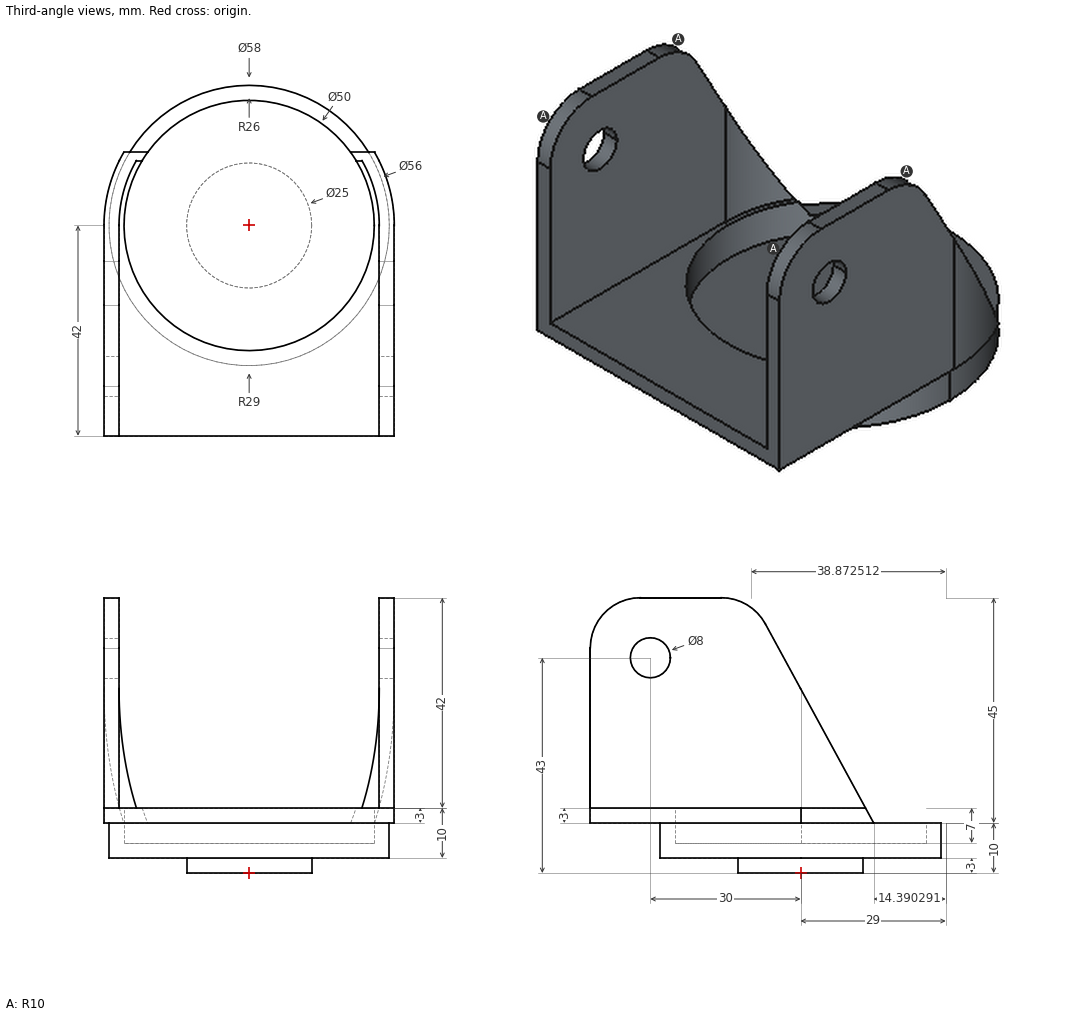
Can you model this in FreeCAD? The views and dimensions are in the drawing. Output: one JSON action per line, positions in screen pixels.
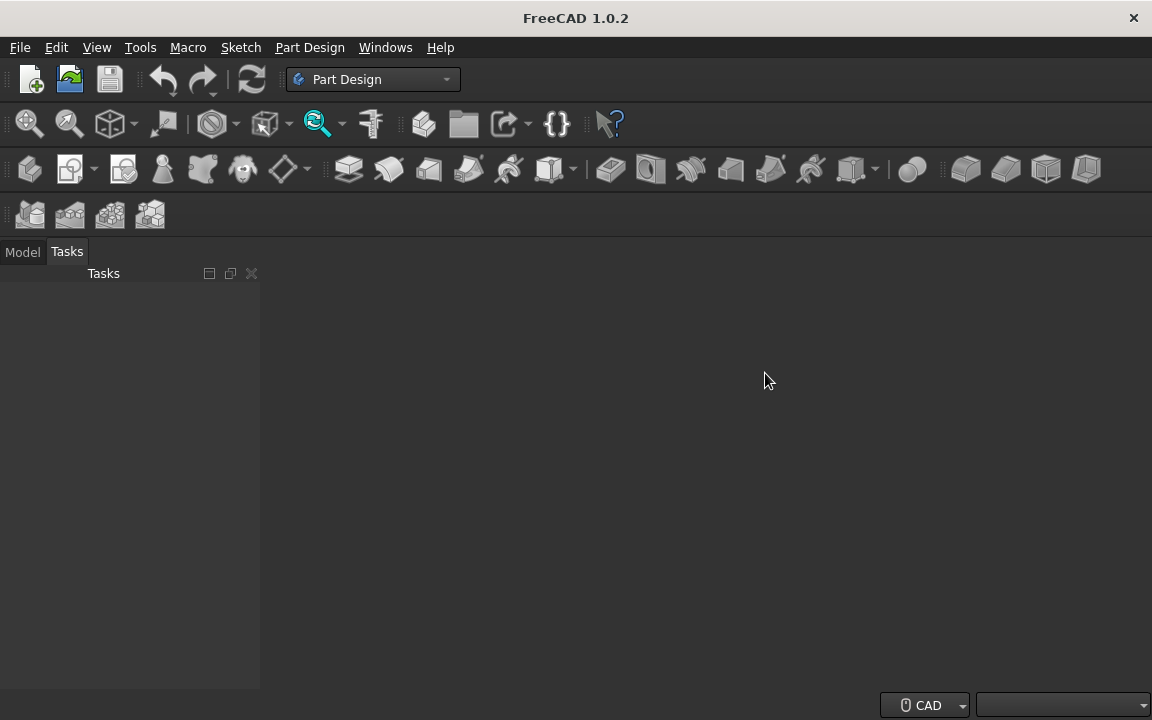
{"action": "left_click", "coordinate": [30, 80]}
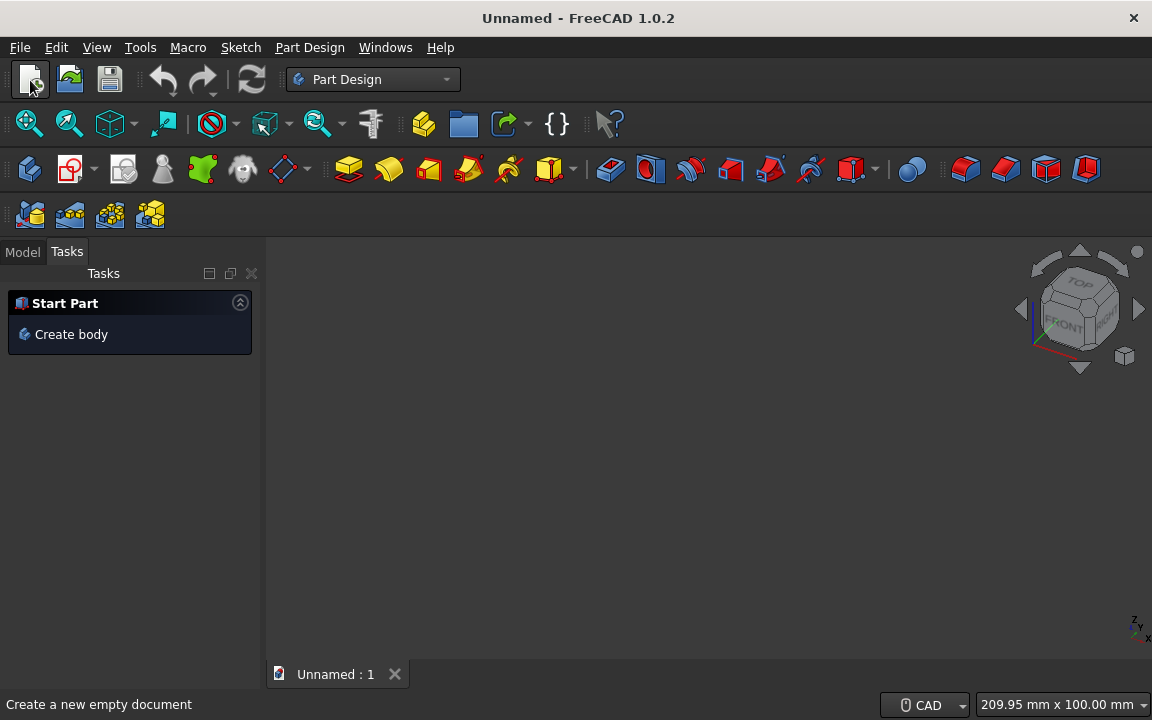
{"action": "left_click", "coordinate": [70, 170]}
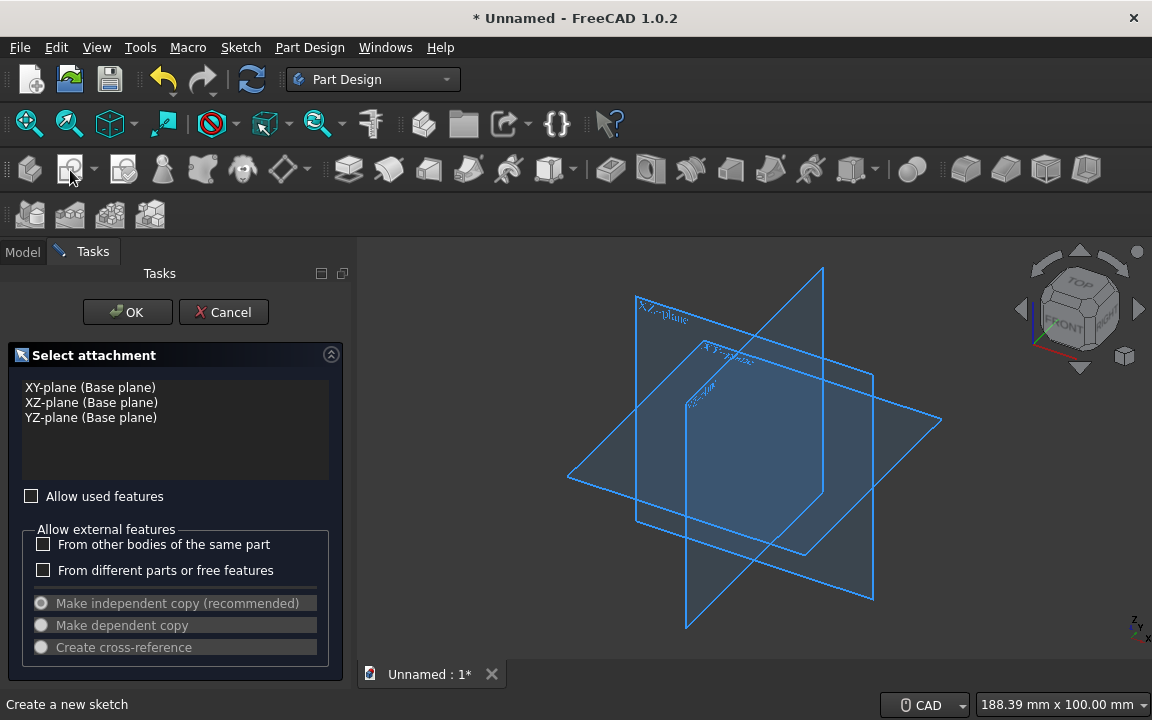
{"action": "left_click", "coordinate": [82, 388]}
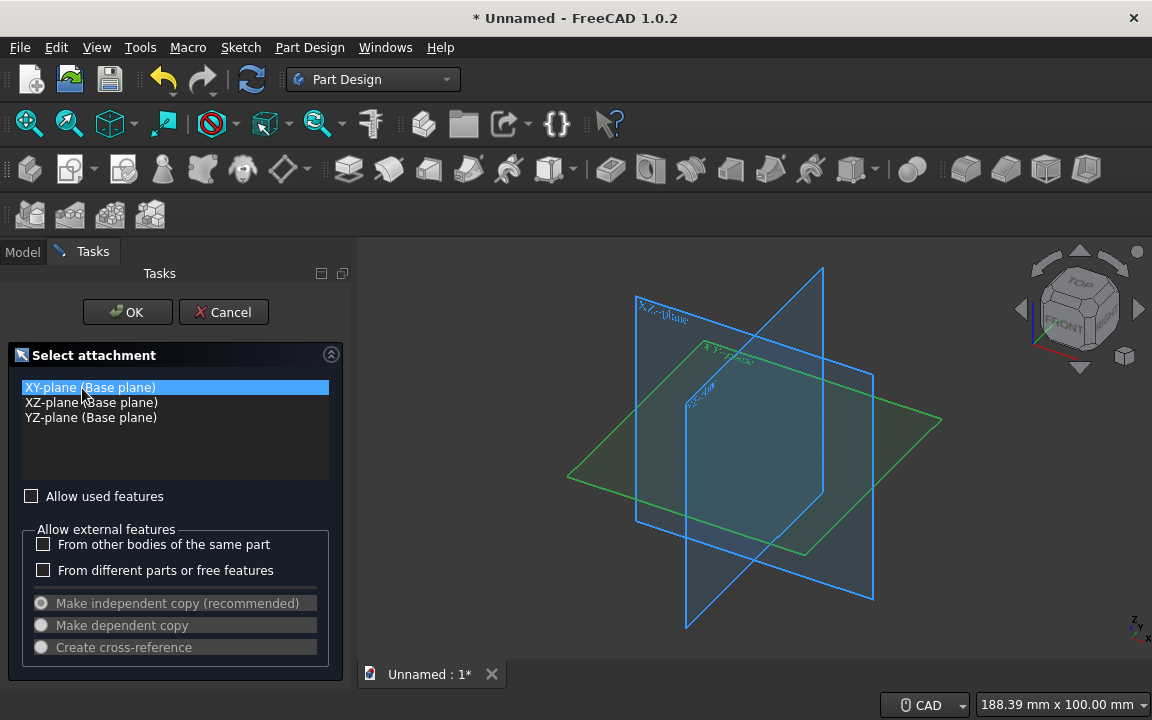
{"action": "left_click", "coordinate": [128, 312]}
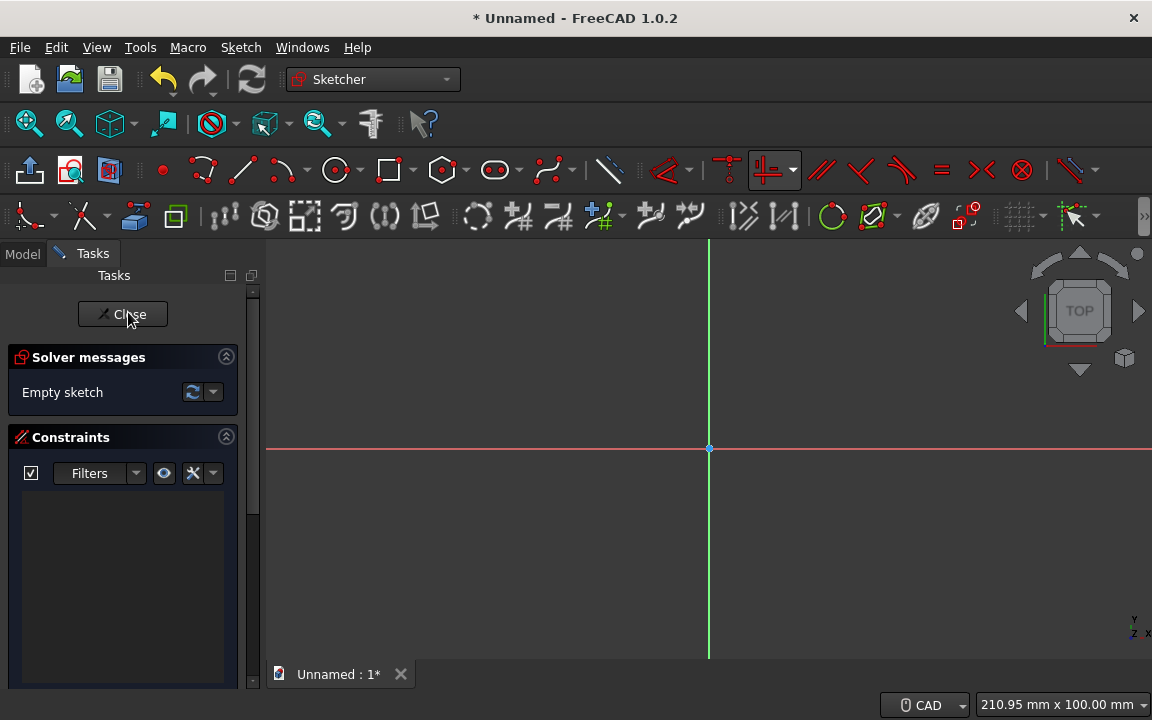
{"action": "scroll", "coordinate": [765, 449], "scroll_direction": "up", "scroll_amount": 4}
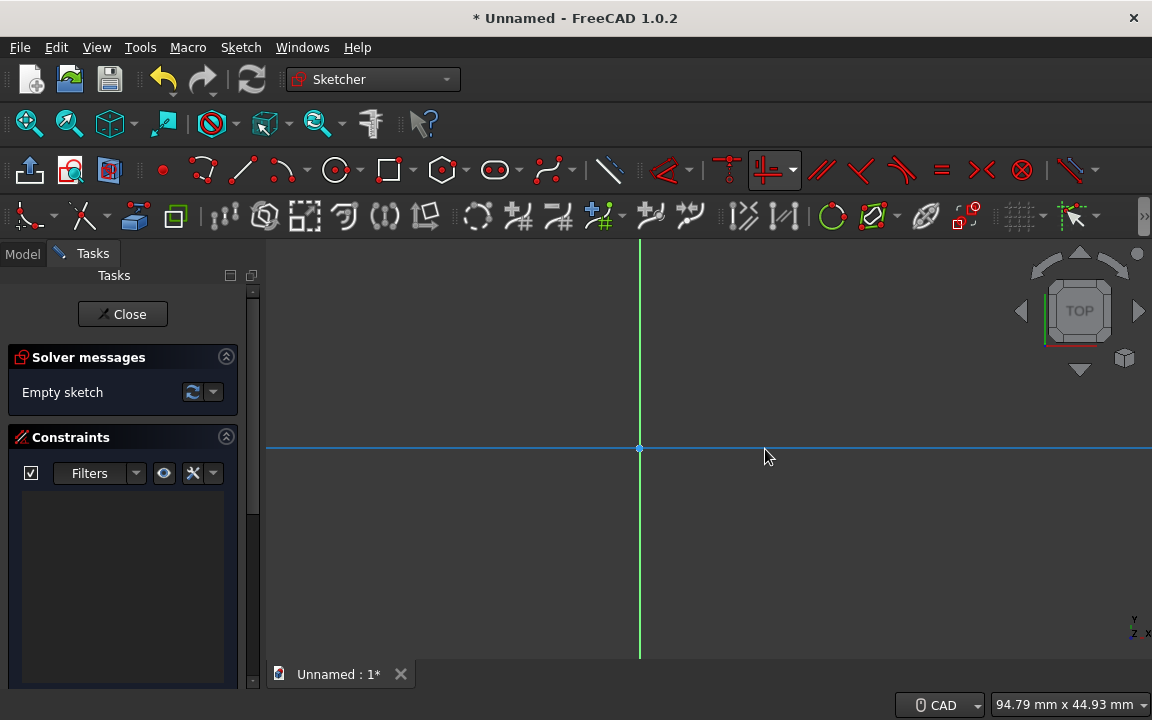
{"action": "left_click", "coordinate": [336, 170]}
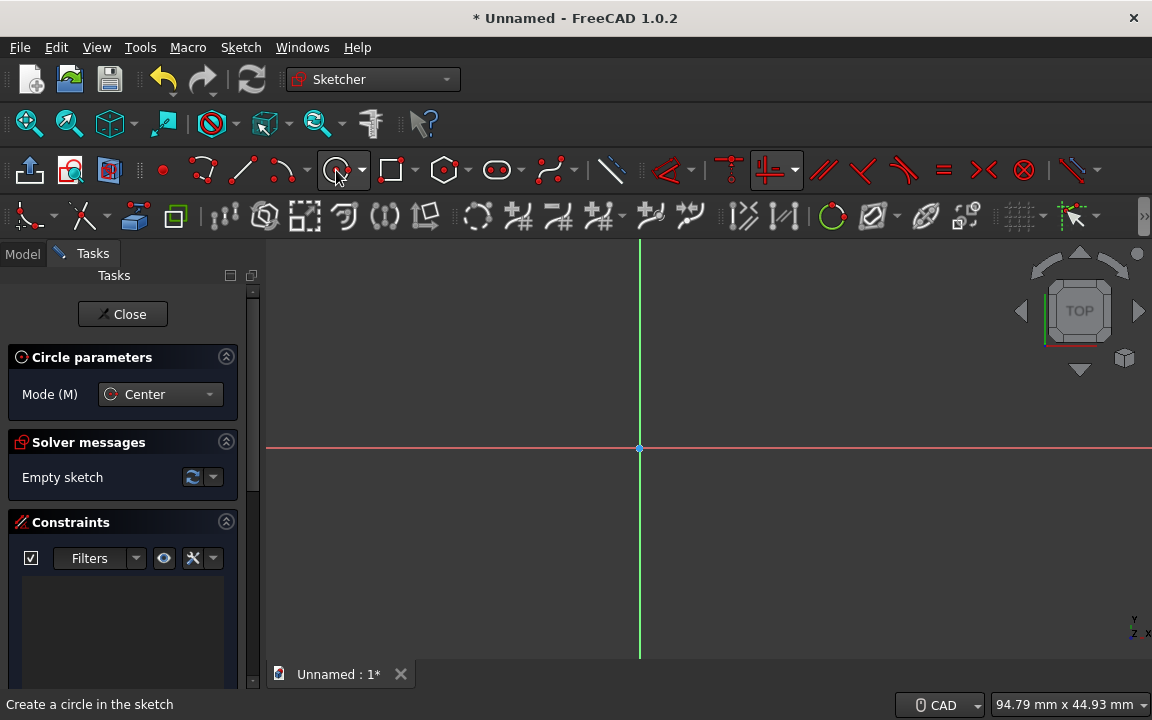
{"action": "left_click", "coordinate": [640, 448]}
{"action": "left_click", "coordinate": [722, 366]}
{"action": "key", "text": "Escape"}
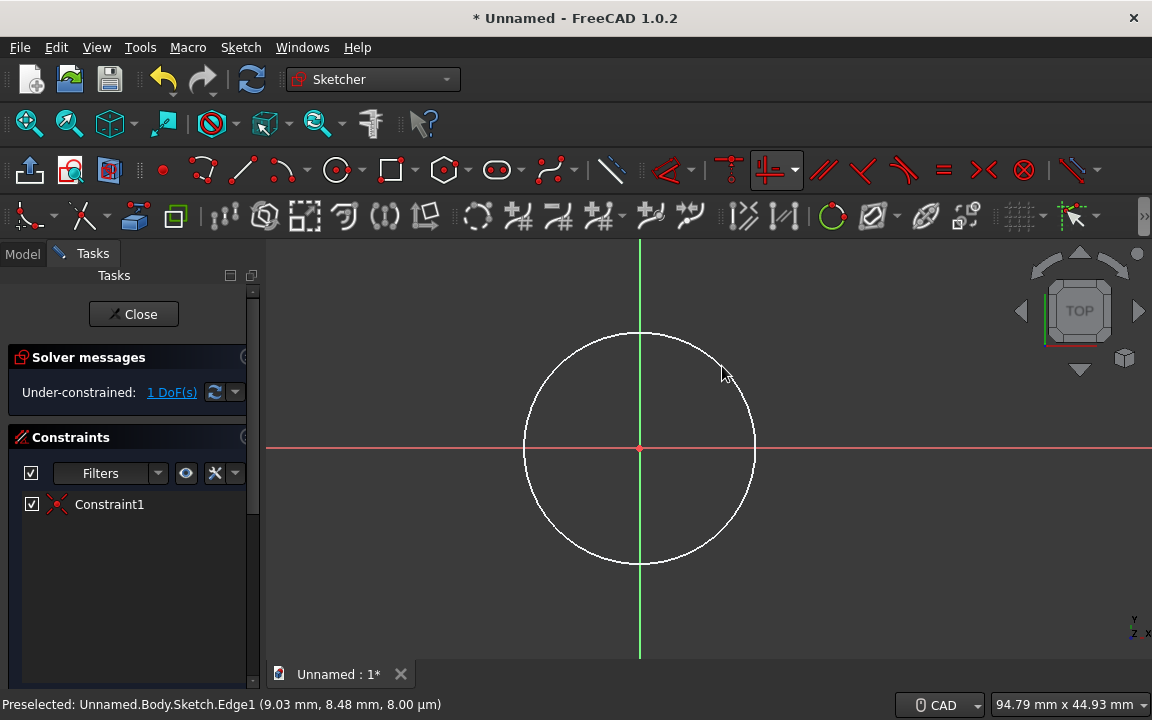
{"action": "left_click", "coordinate": [666, 170]}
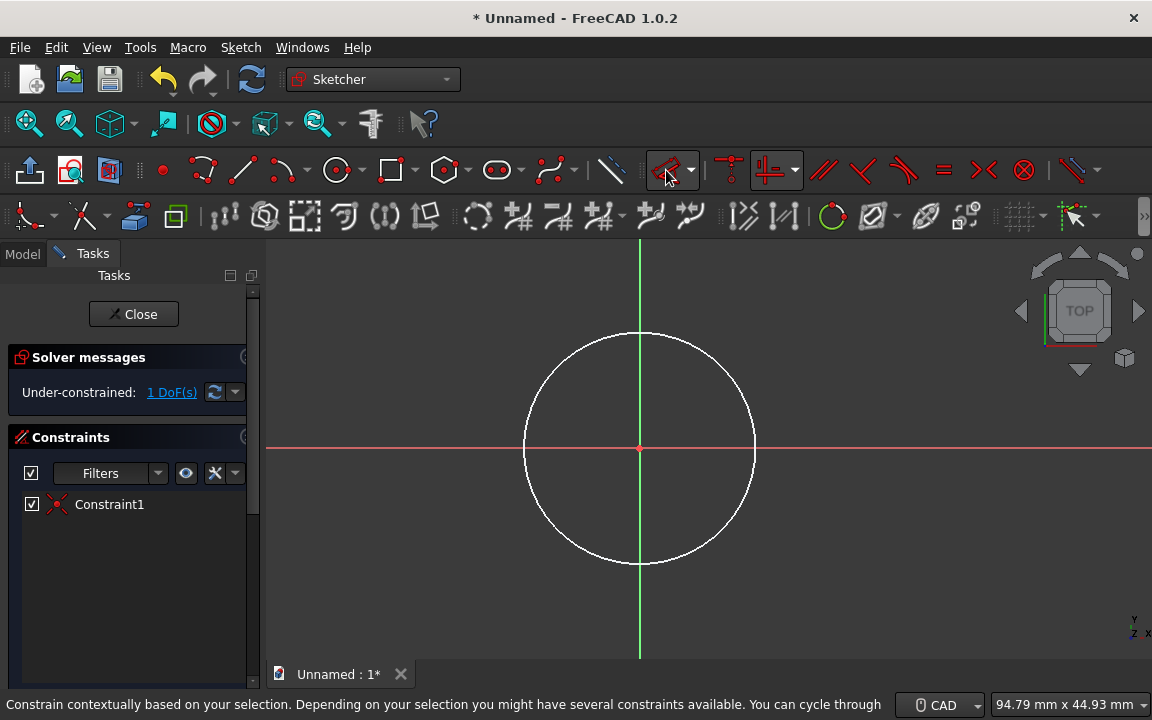
{"action": "left_click", "coordinate": [721, 366]}
{"action": "left_click", "coordinate": [743, 343]}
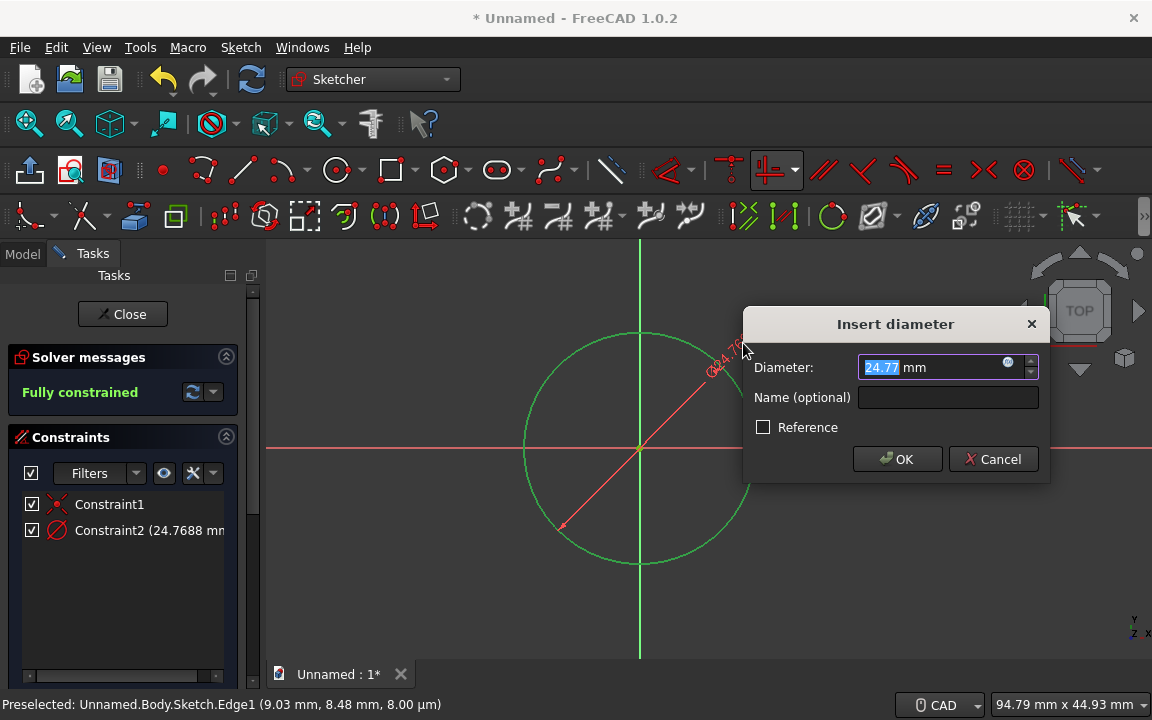
{"action": "type", "text": "25"}
{"action": "key", "text": "Return"}
{"action": "key", "text": "Escape"}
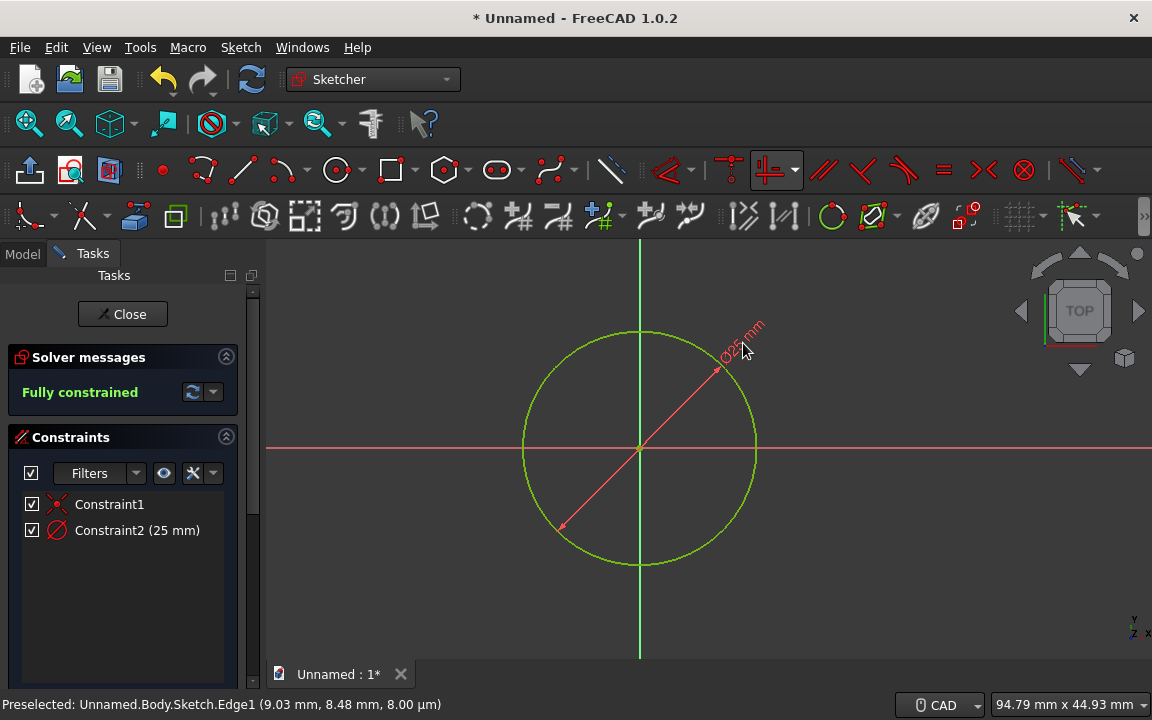
{"action": "left_click", "coordinate": [123, 314]}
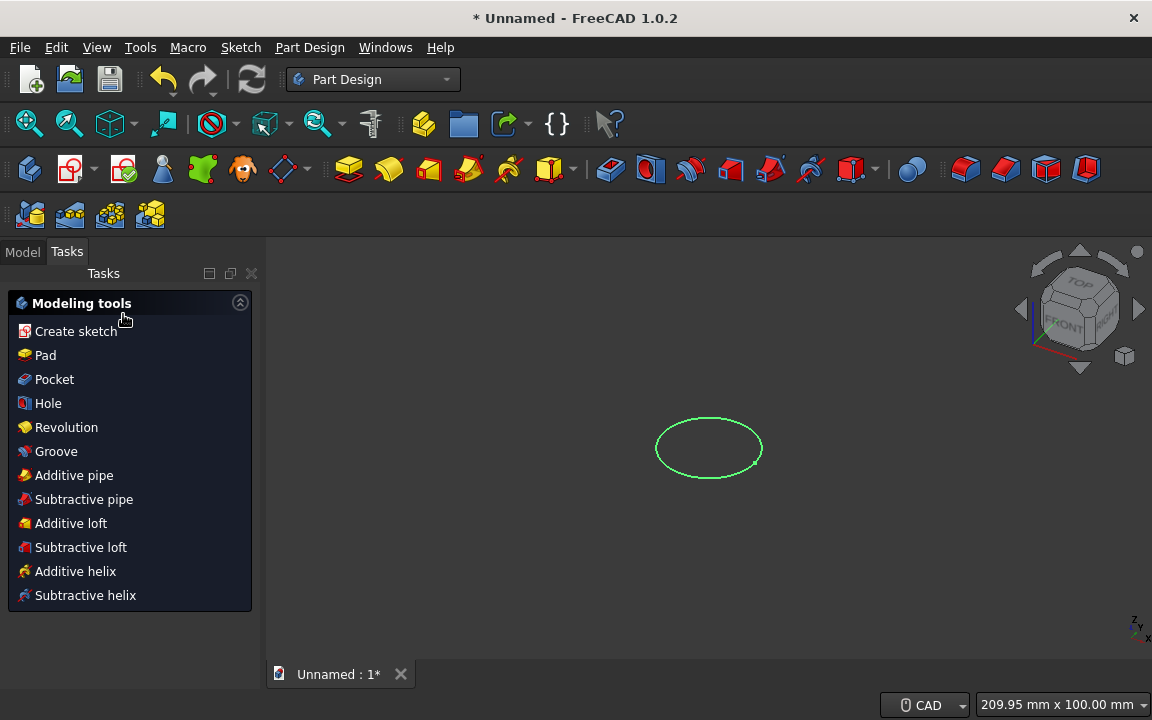
{"action": "left_click", "coordinate": [350, 170]}